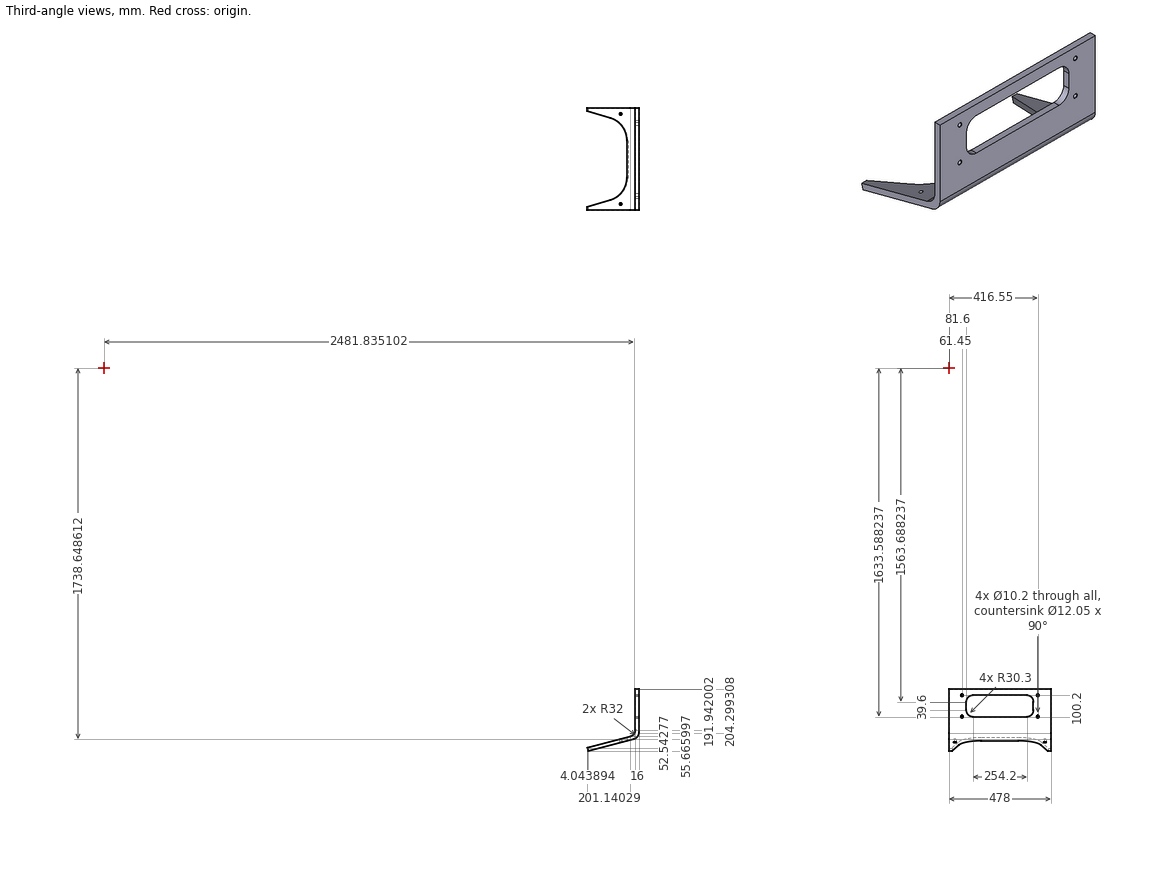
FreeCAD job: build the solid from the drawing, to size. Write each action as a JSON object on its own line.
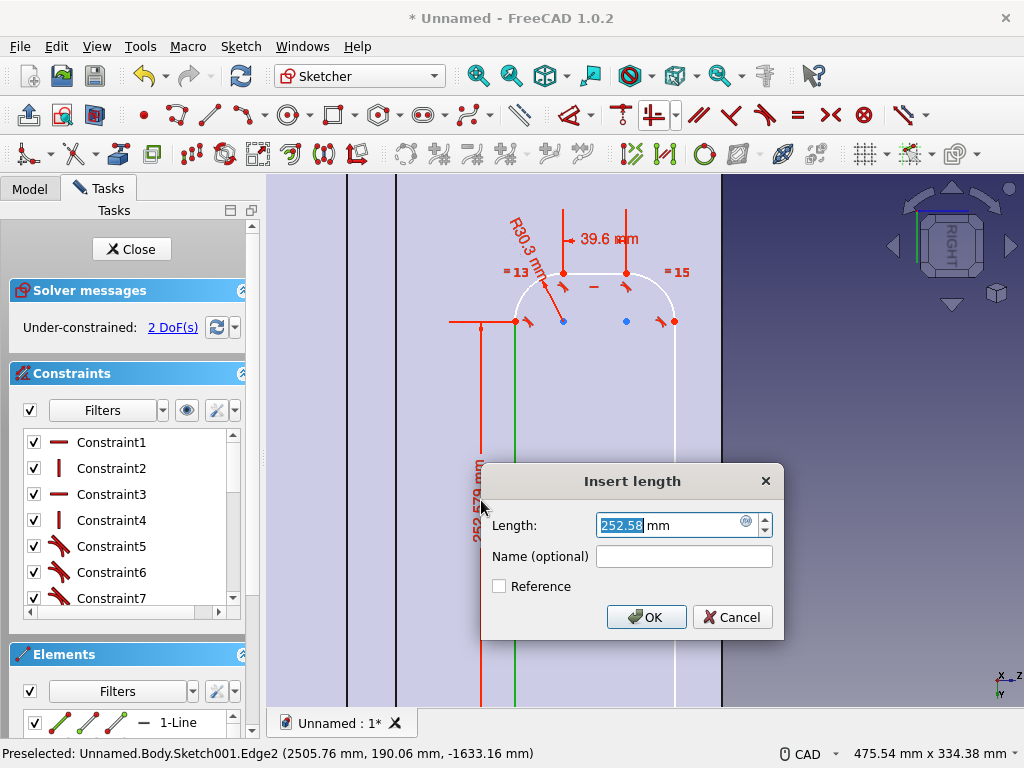
{"action": "type", "text": "254.2"}
{"action": "key", "text": "Return"}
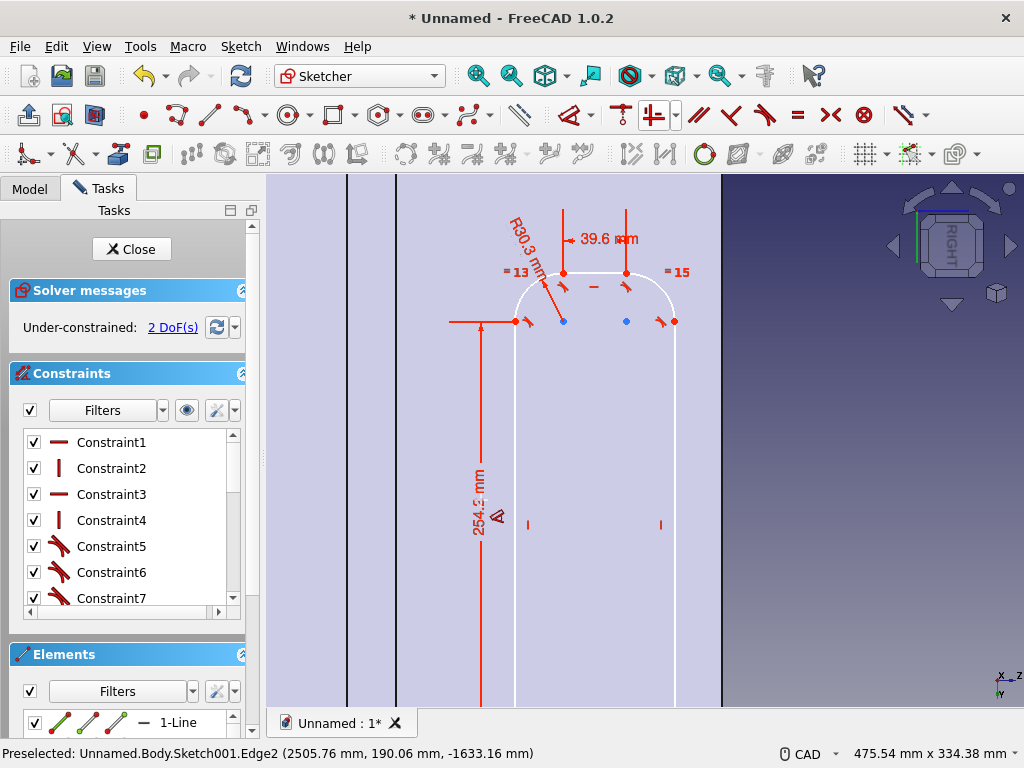
{"action": "left_click", "coordinate": [626, 273]}
{"action": "left_click", "coordinate": [592, 213]}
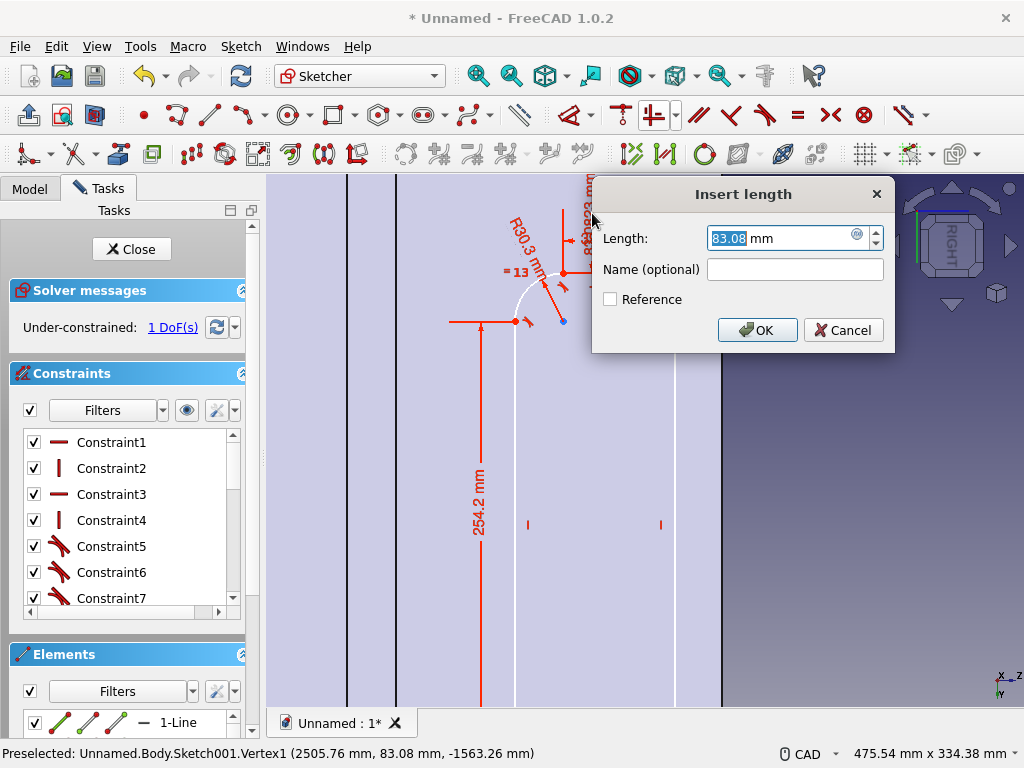
{"action": "type", "text": "81.6"}
{"action": "key", "text": "Return"}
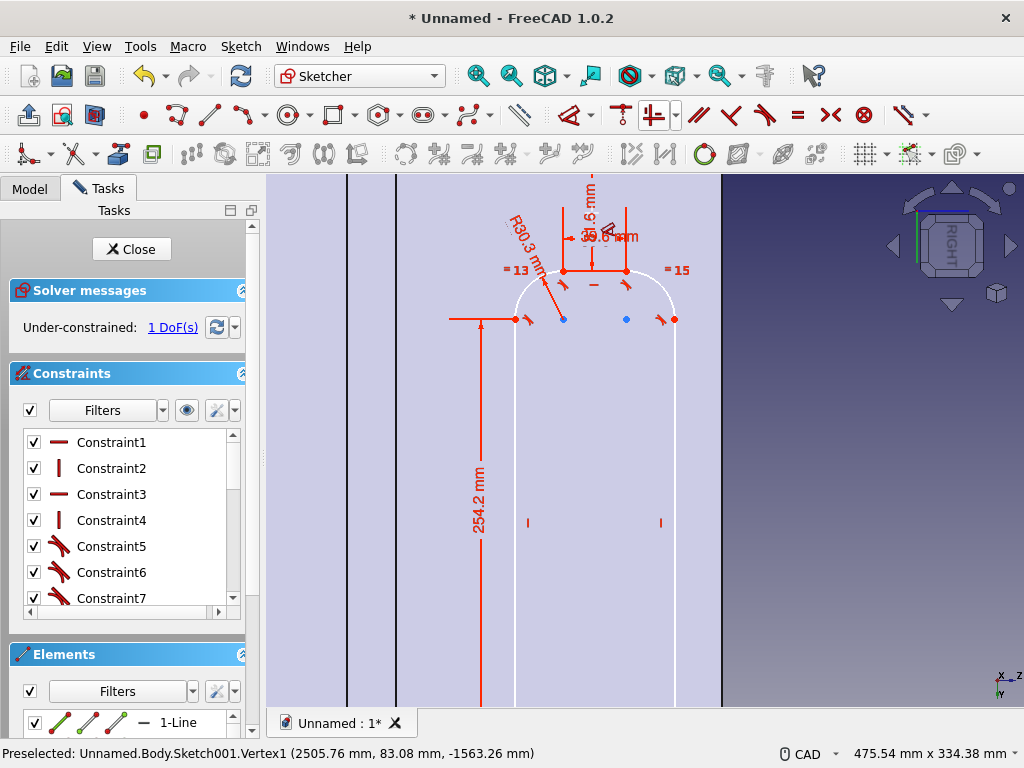
{"action": "left_click", "coordinate": [626, 271]}
{"action": "left_click", "coordinate": [743, 305]}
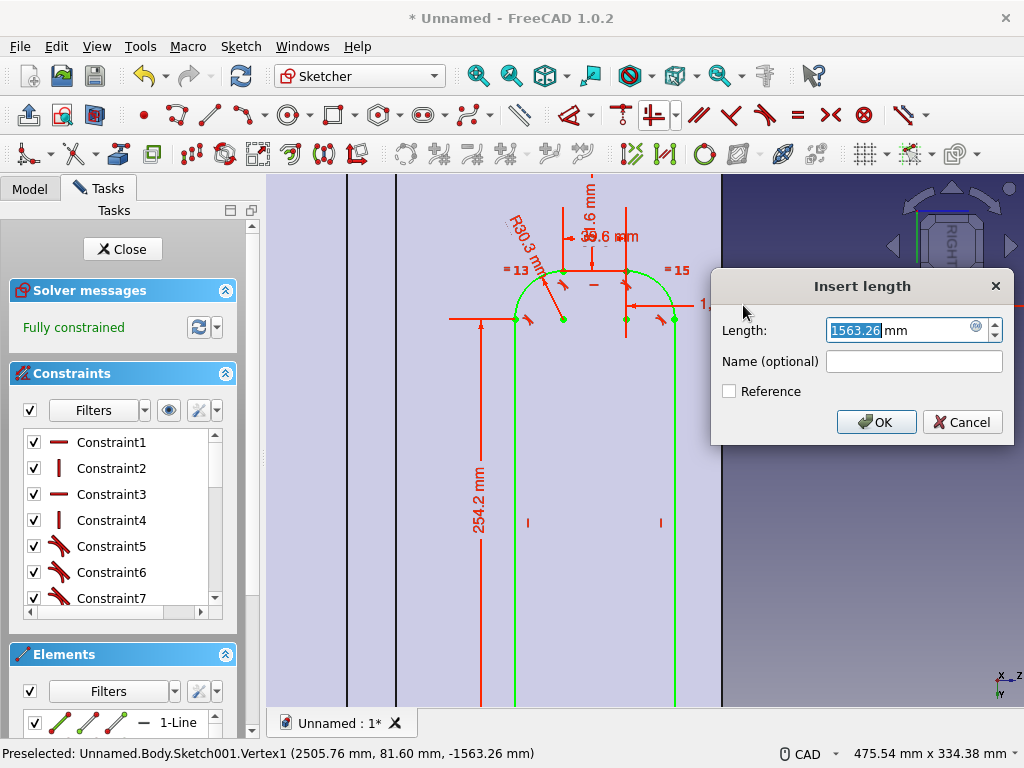
{"action": "type", "text": "1563.688237"}
{"action": "key", "text": "Return"}
{"action": "key", "text": "Escape"}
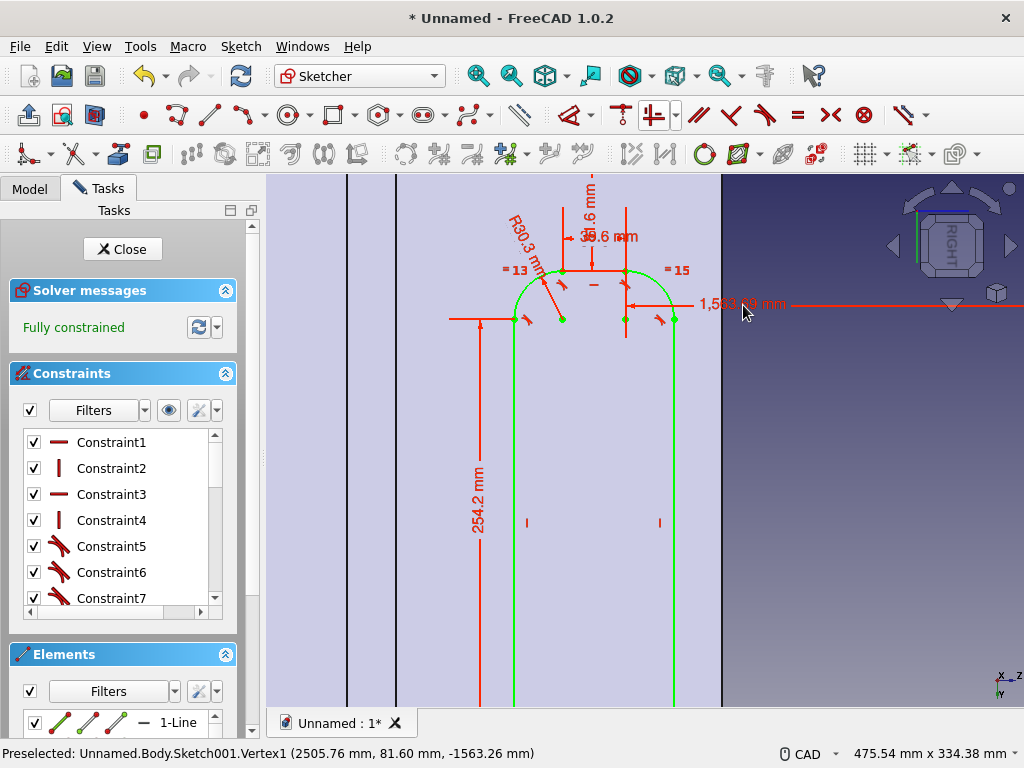
{"action": "left_click", "coordinate": [123, 249]}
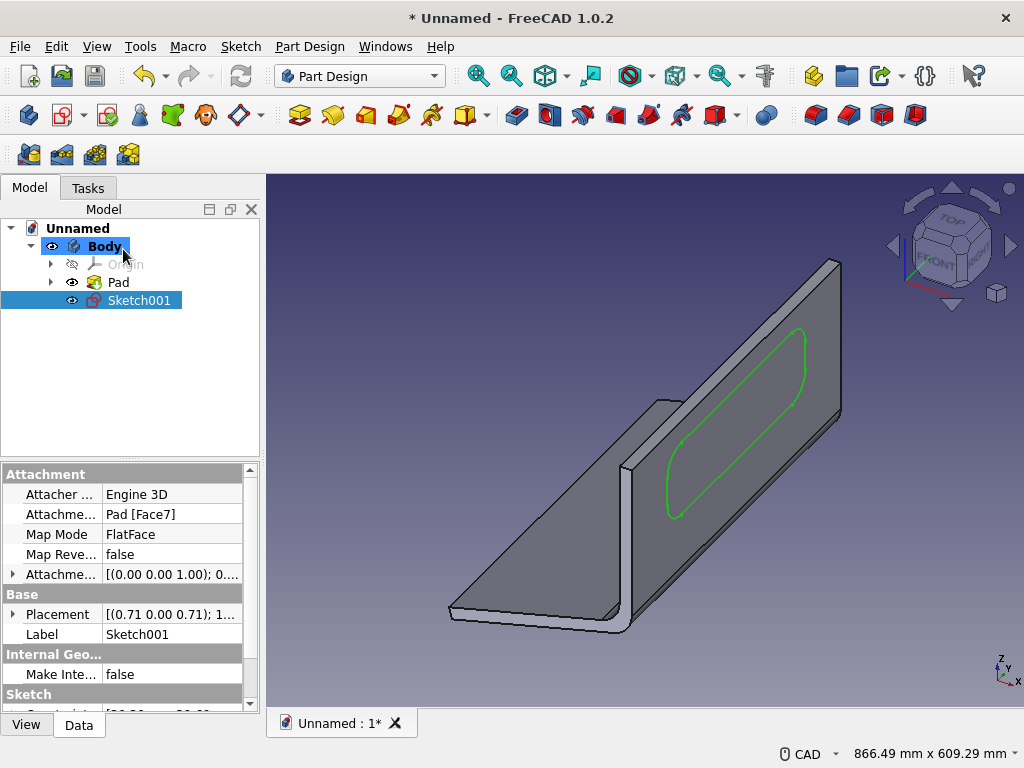
{"action": "left_click", "coordinate": [517, 116]}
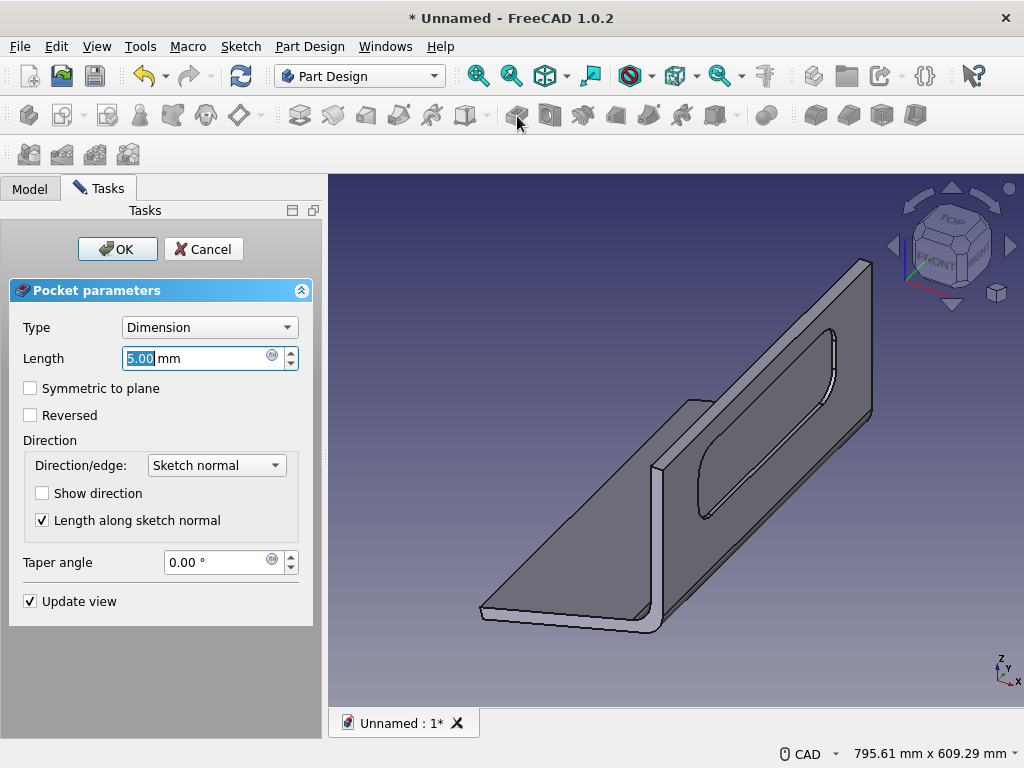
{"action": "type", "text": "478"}
{"action": "key", "text": "Tab"}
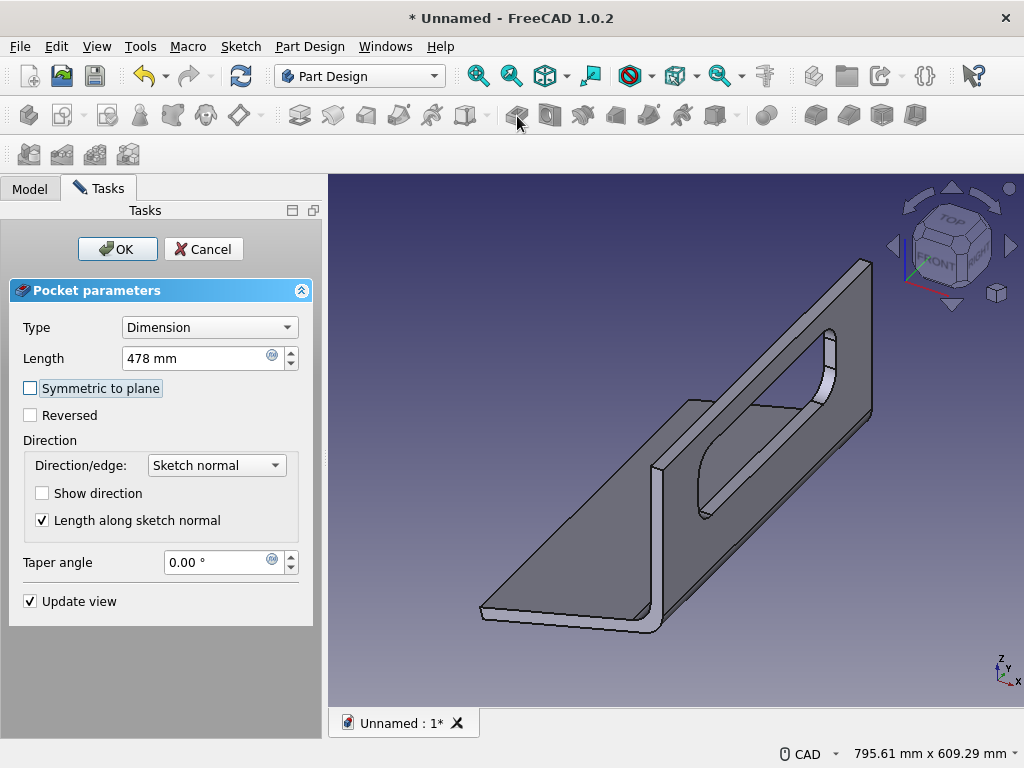
{"action": "left_click", "coordinate": [118, 249]}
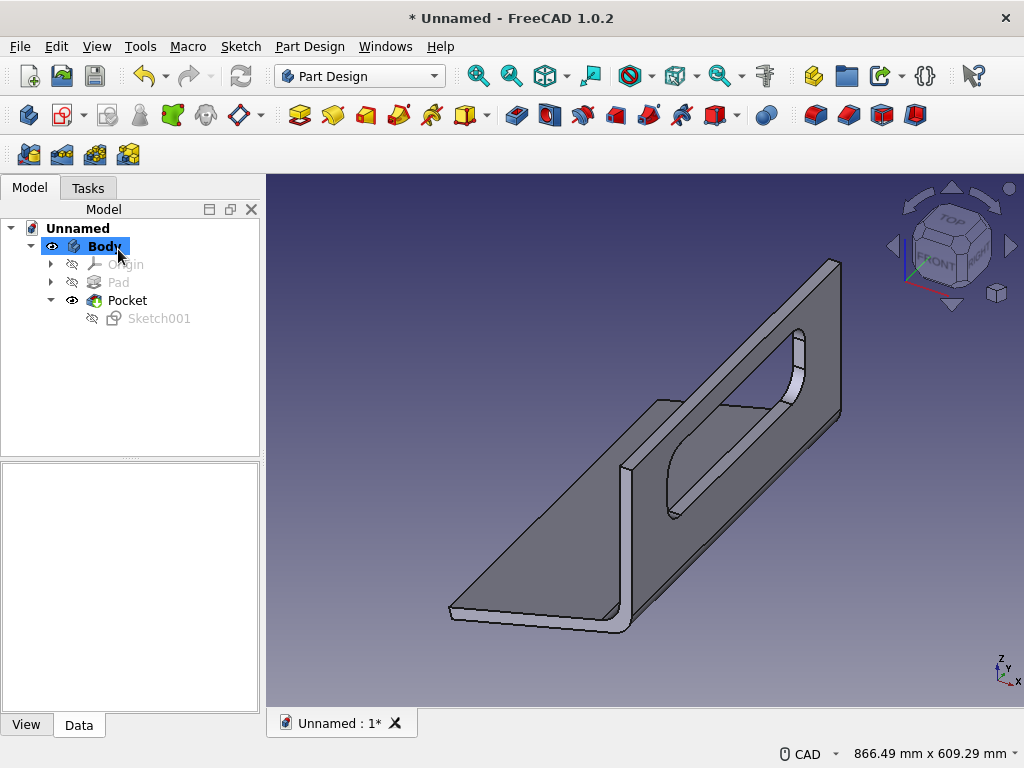
{"action": "left_click", "coordinate": [826, 329]}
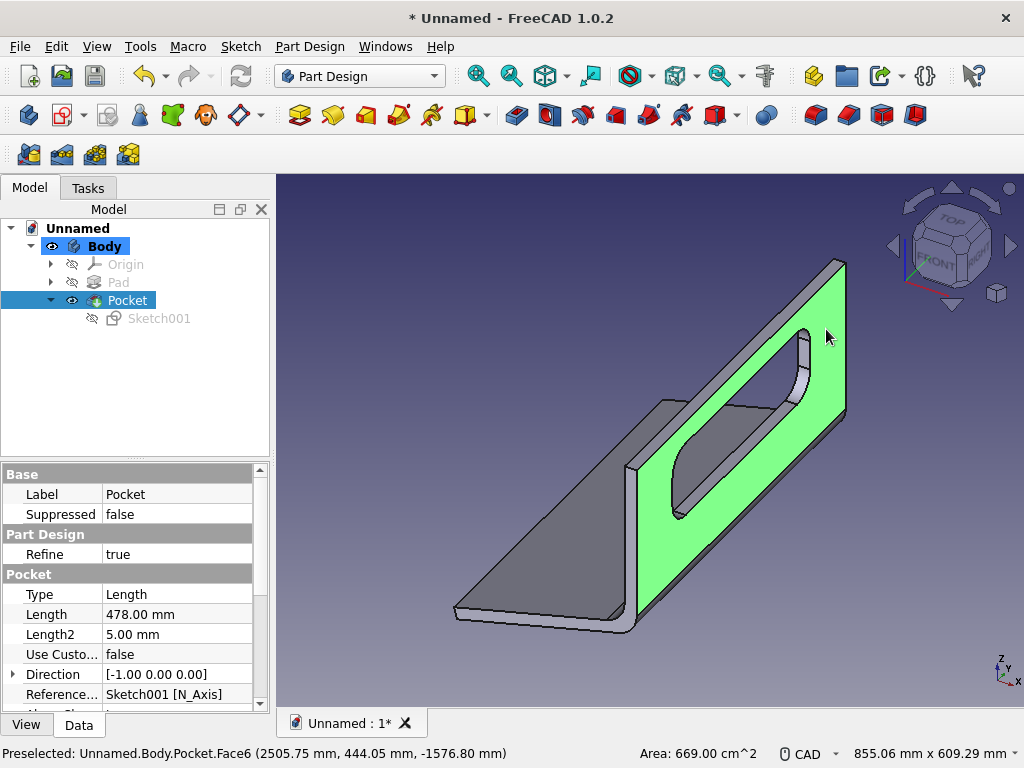
{"action": "left_click", "coordinate": [62, 116]}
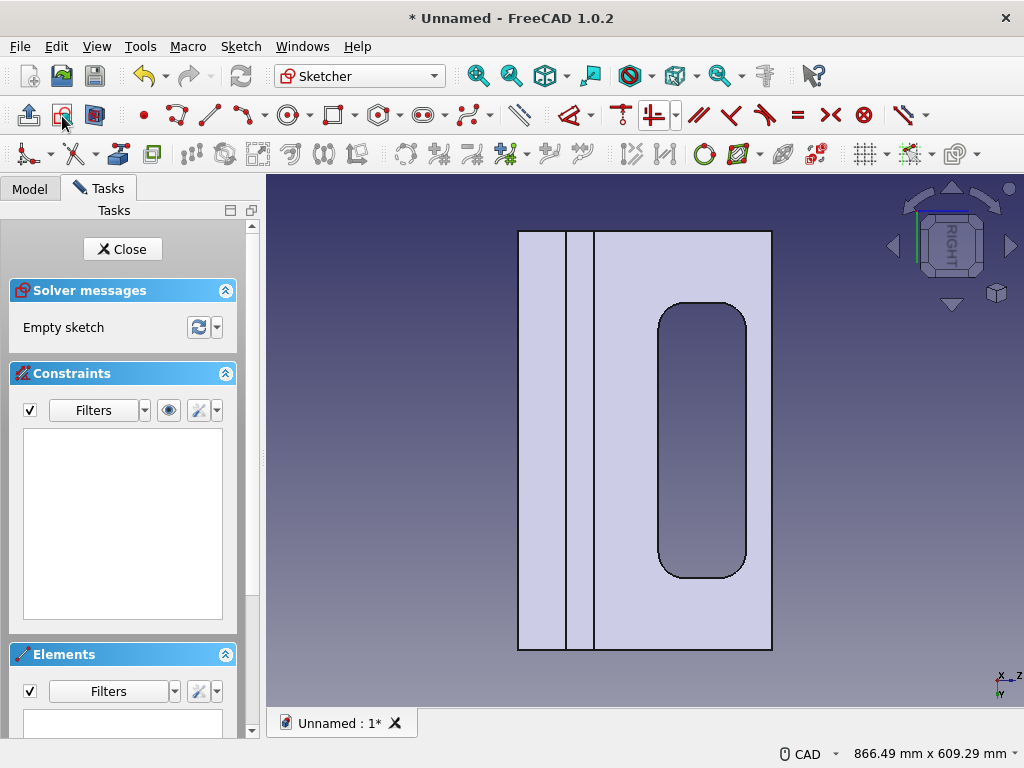
{"action": "left_click", "coordinate": [288, 116]}